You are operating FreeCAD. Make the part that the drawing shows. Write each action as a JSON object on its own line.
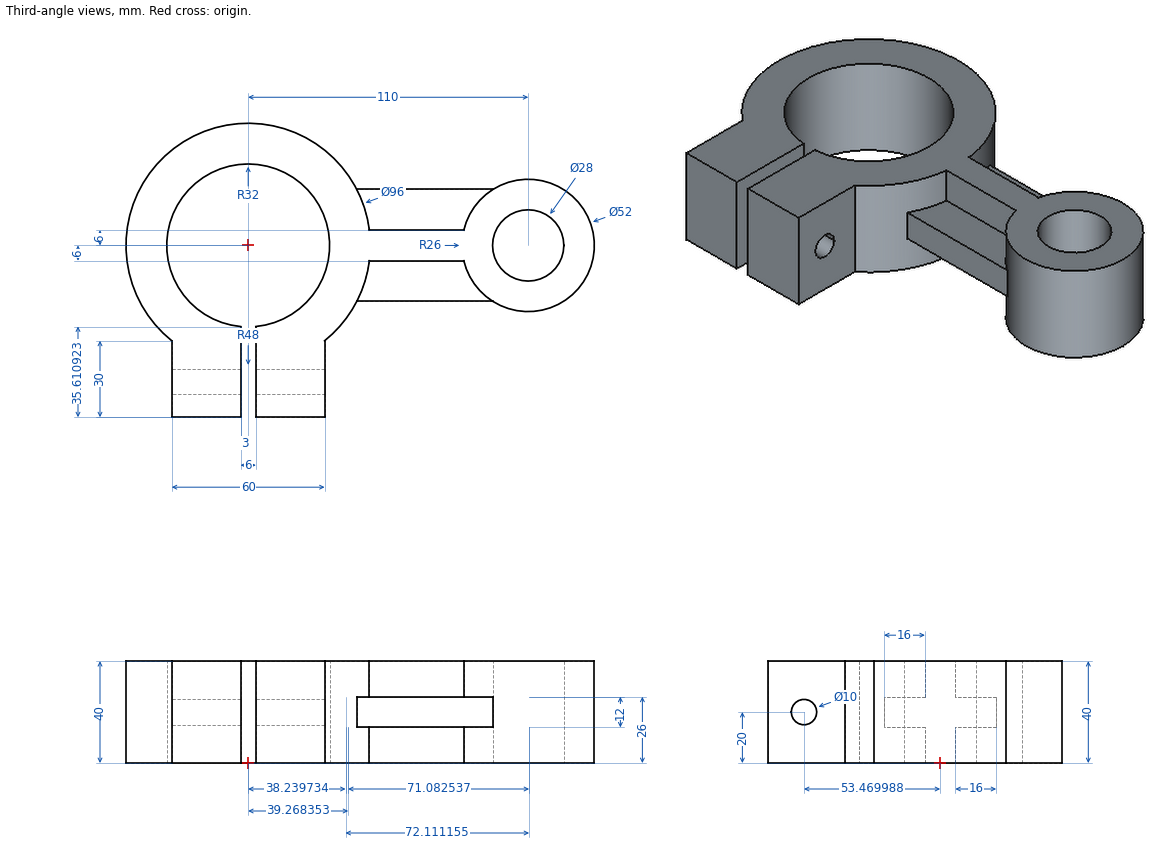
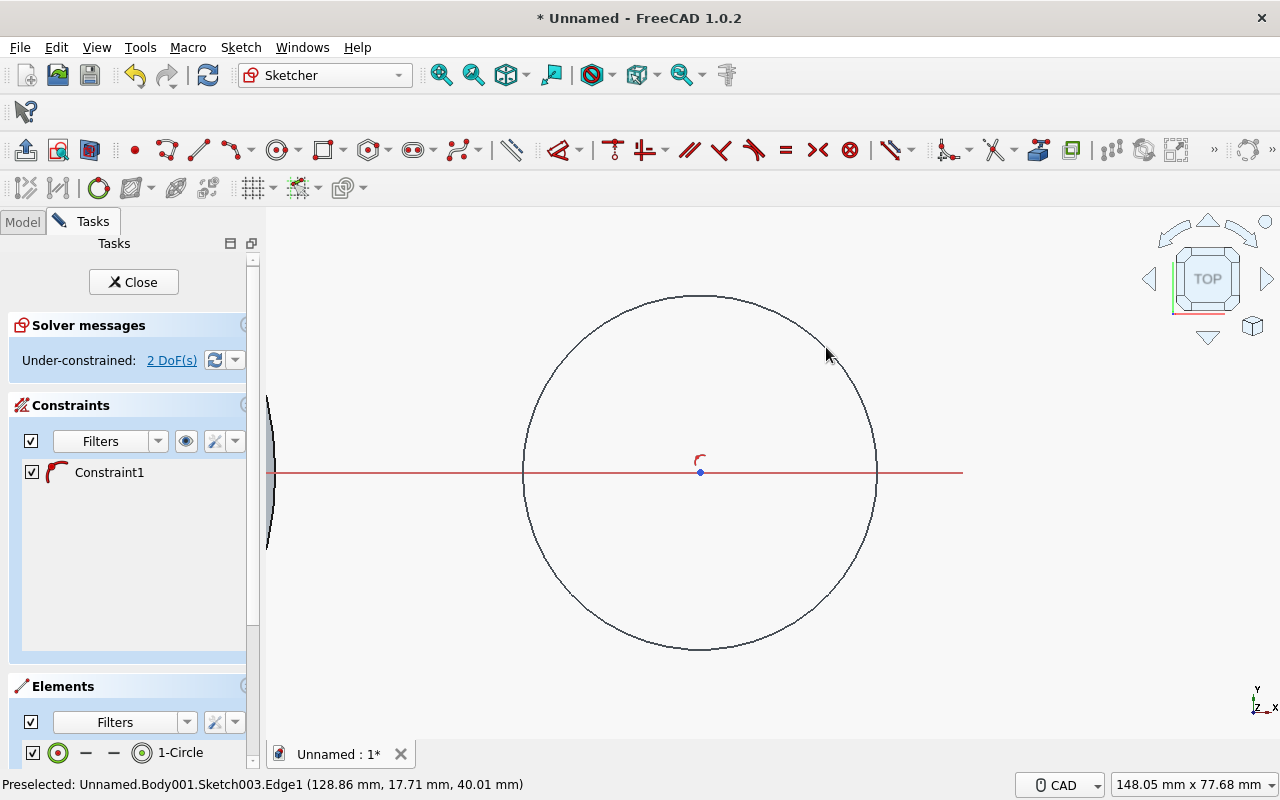
{"action": "left_click", "coordinate": [558, 150]}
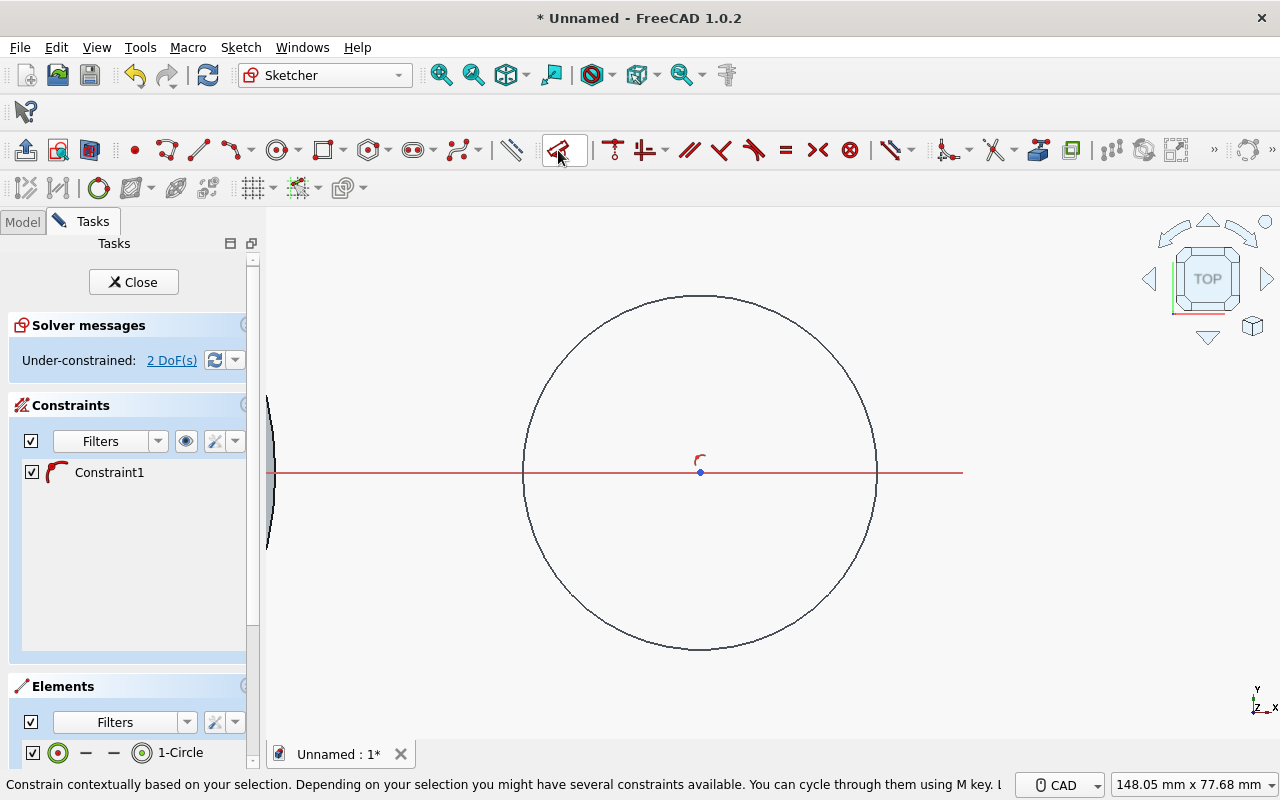
{"action": "left_click", "coordinate": [825, 347]}
{"action": "left_click", "coordinate": [848, 324]}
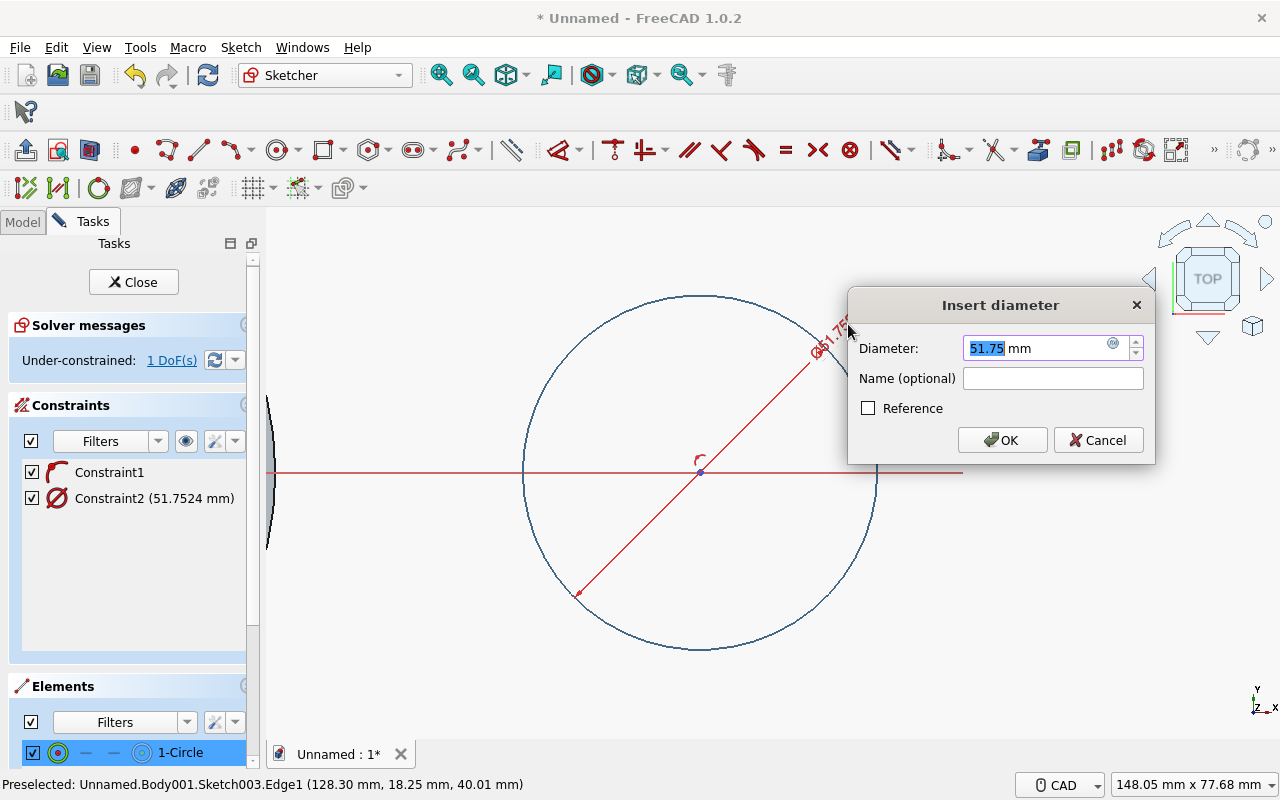
{"action": "type", "text": "52"}
{"action": "key", "text": "Return"}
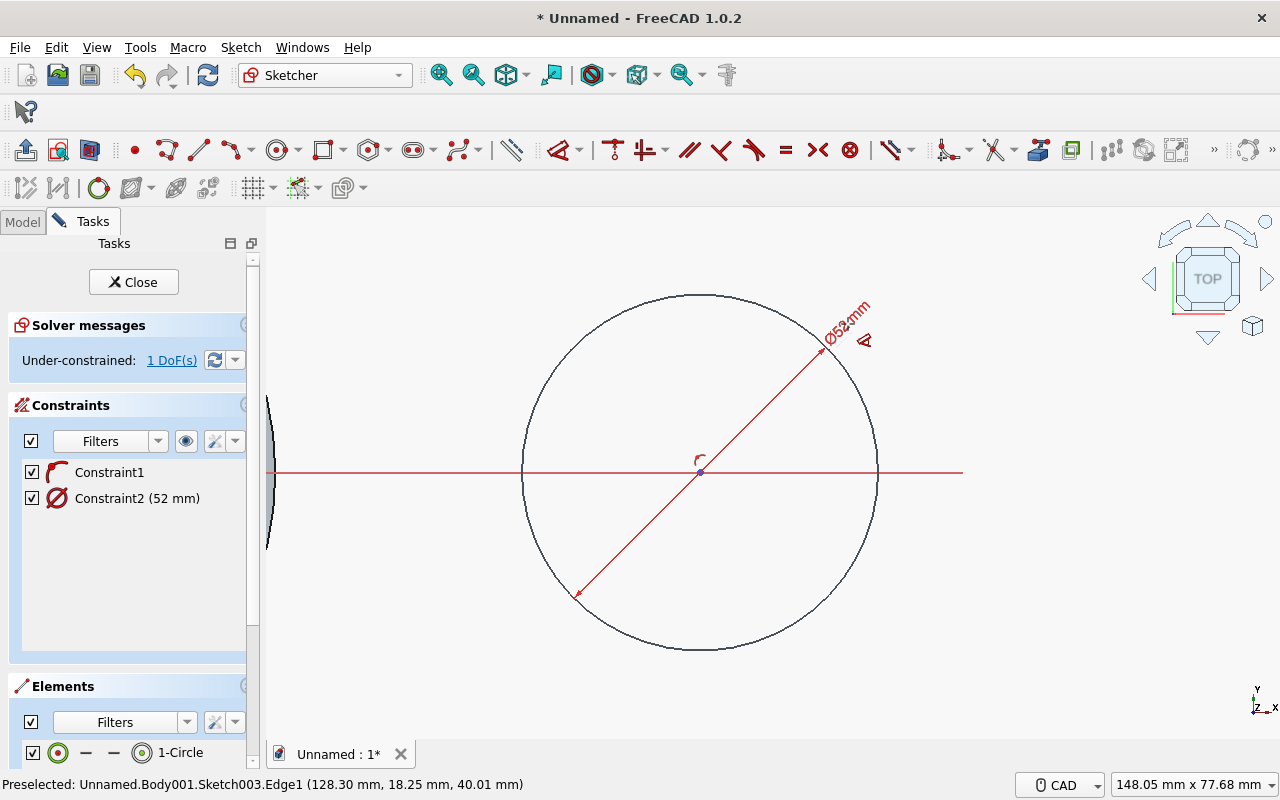
{"action": "left_click", "coordinate": [700, 473]}
{"action": "left_click", "coordinate": [497, 507]}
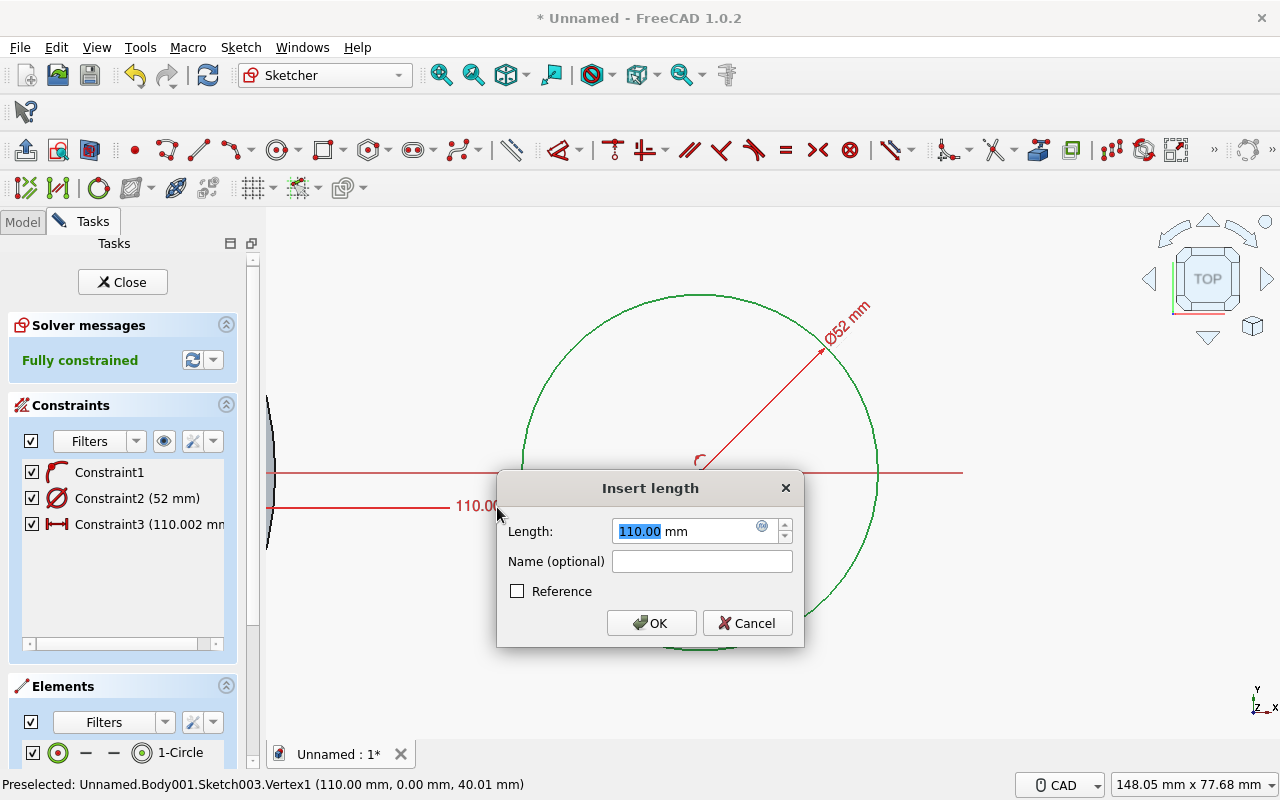
{"action": "type", "text": "110"}
{"action": "key", "text": "Return"}
{"action": "key", "text": "Escape"}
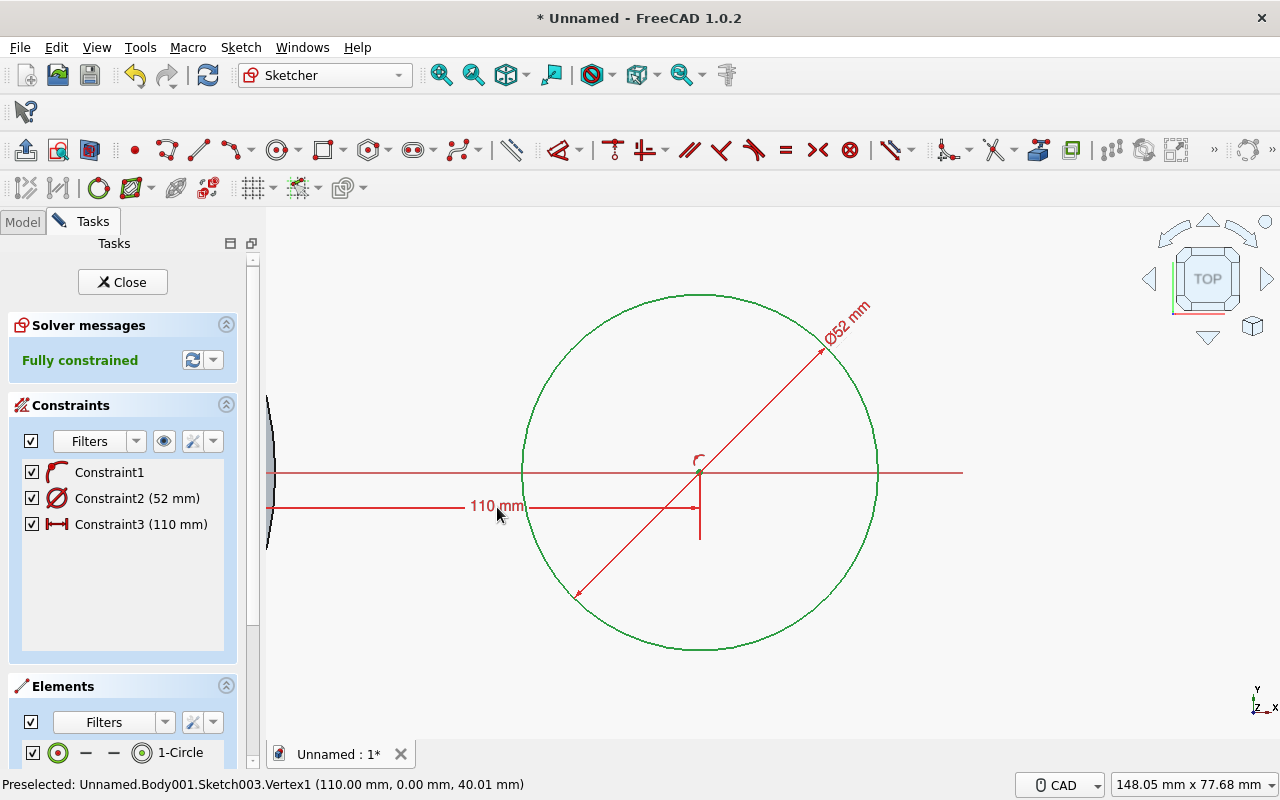
{"action": "left_click", "coordinate": [123, 282]}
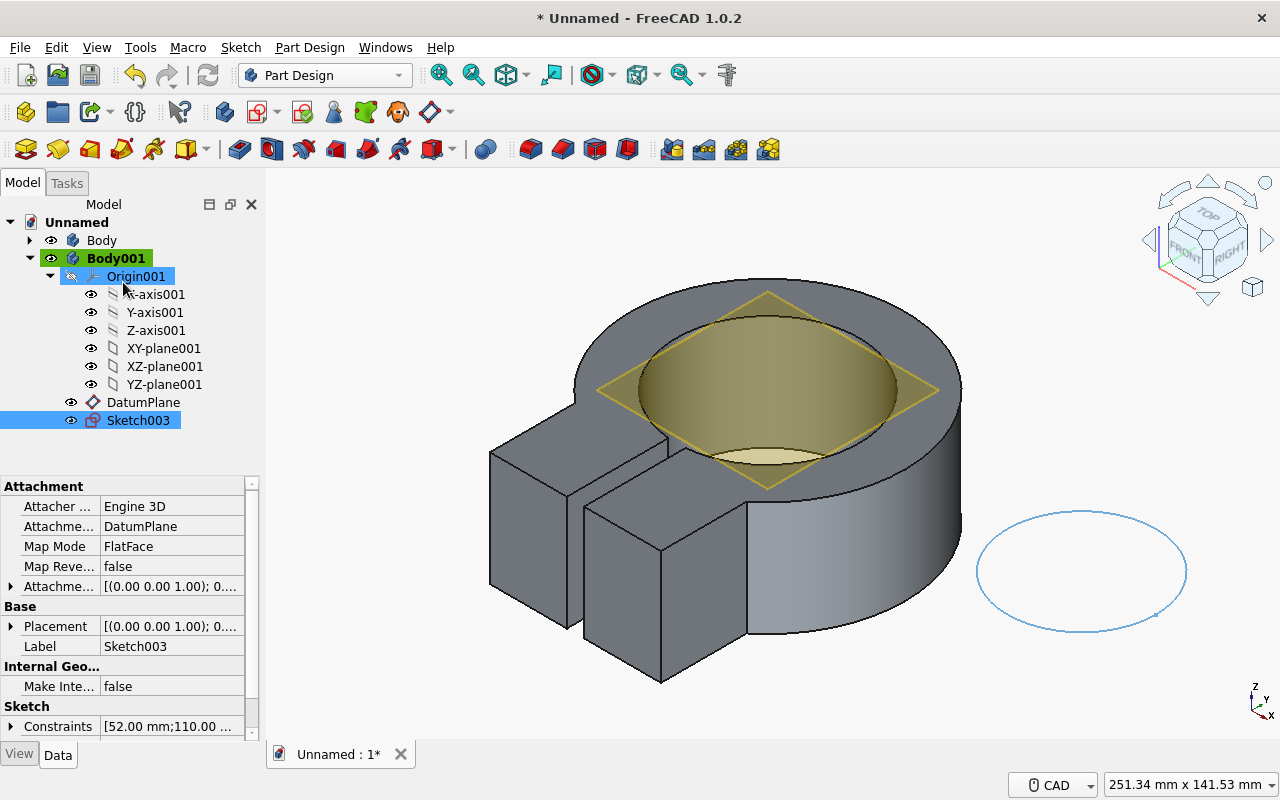
{"action": "left_click", "coordinate": [26, 150]}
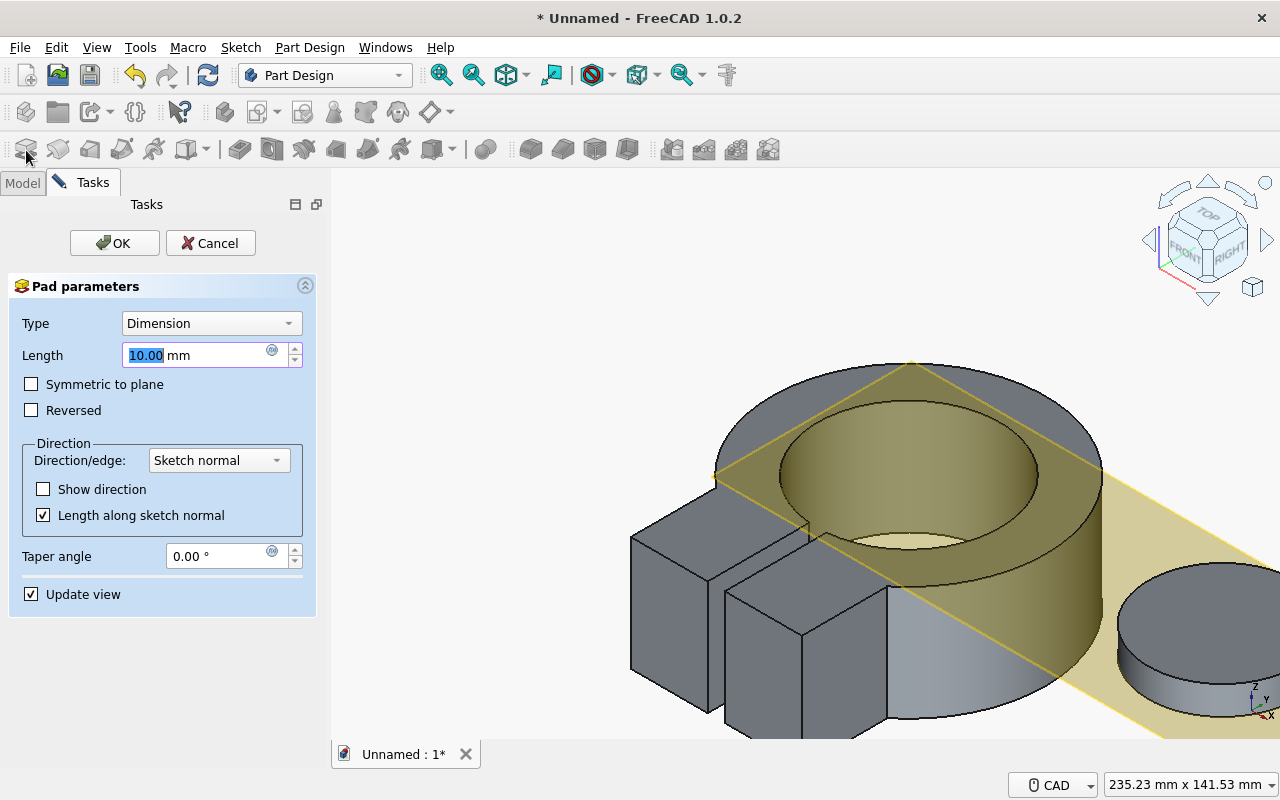
{"action": "type", "text": "40"}
{"action": "key", "text": "Tab"}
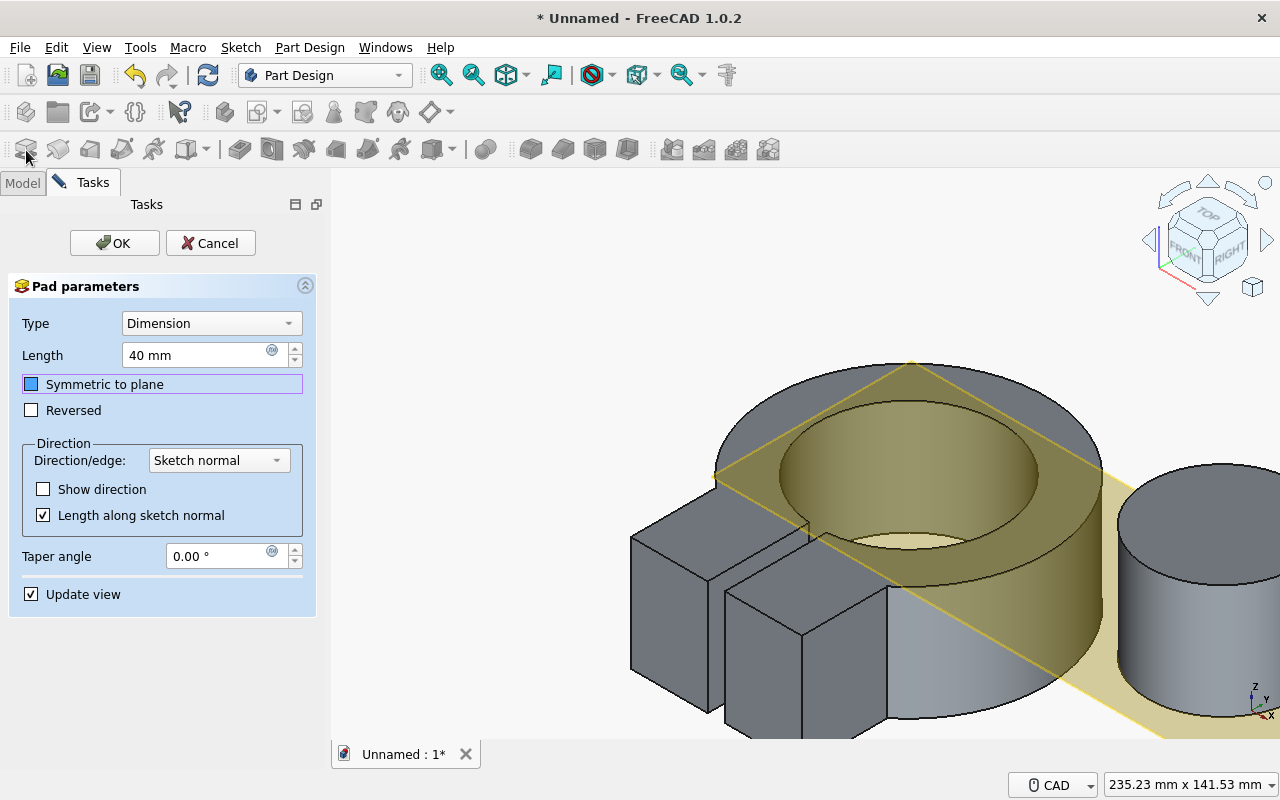
{"action": "left_click", "coordinate": [30, 410]}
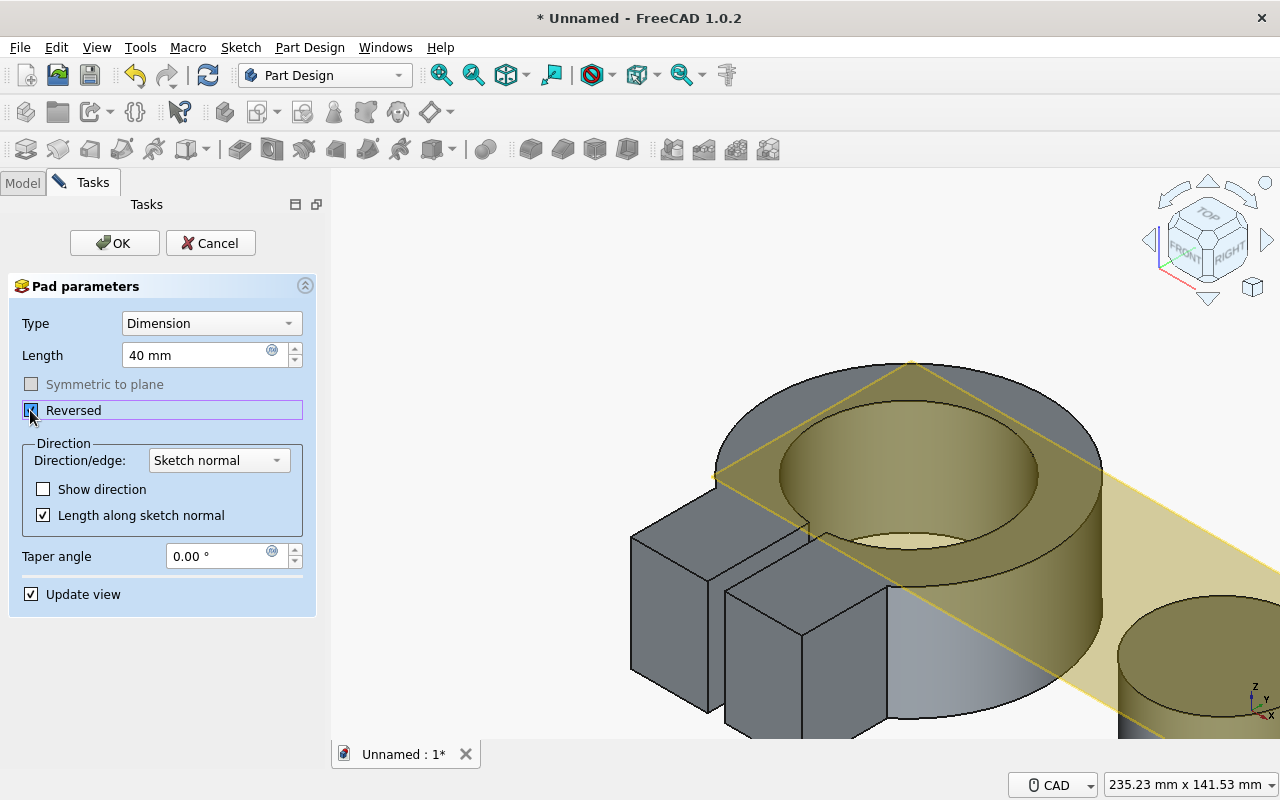
{"action": "left_click", "coordinate": [115, 243]}